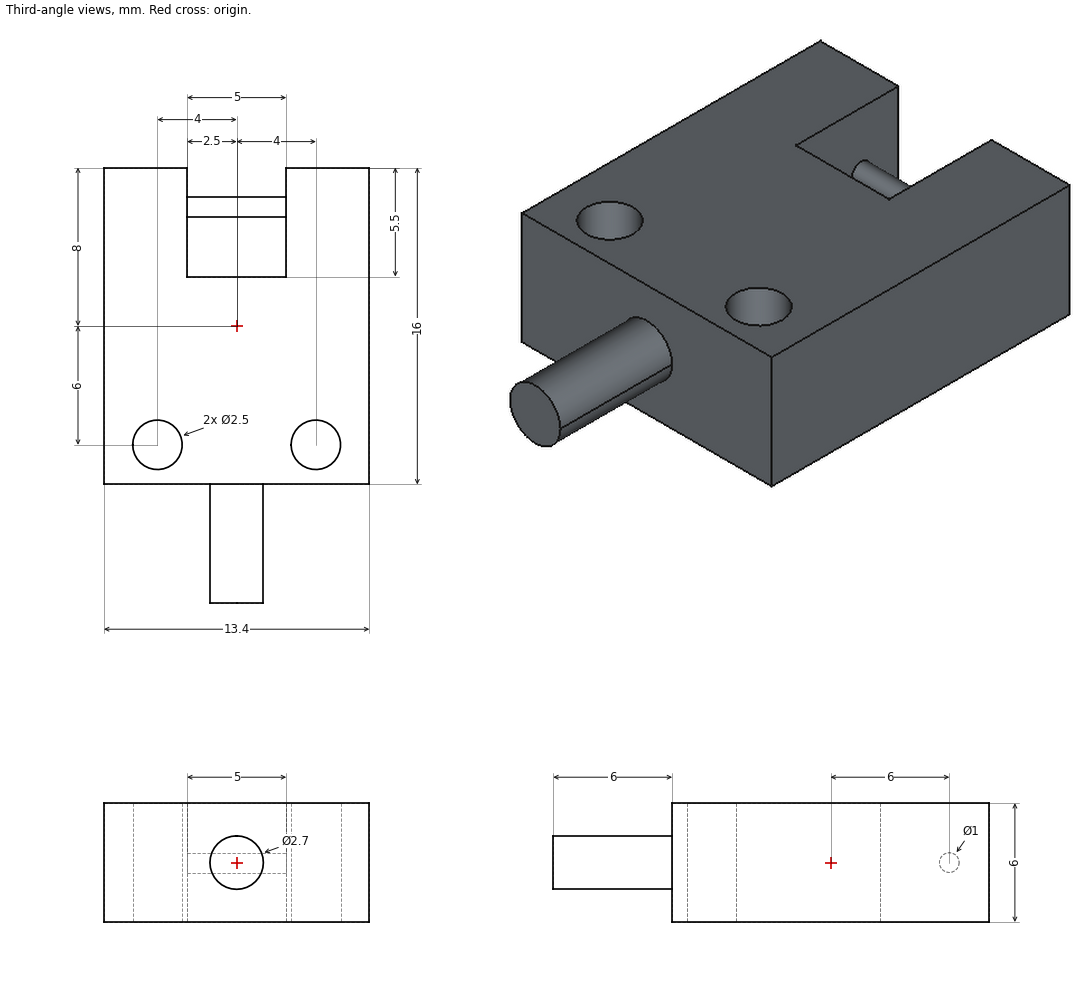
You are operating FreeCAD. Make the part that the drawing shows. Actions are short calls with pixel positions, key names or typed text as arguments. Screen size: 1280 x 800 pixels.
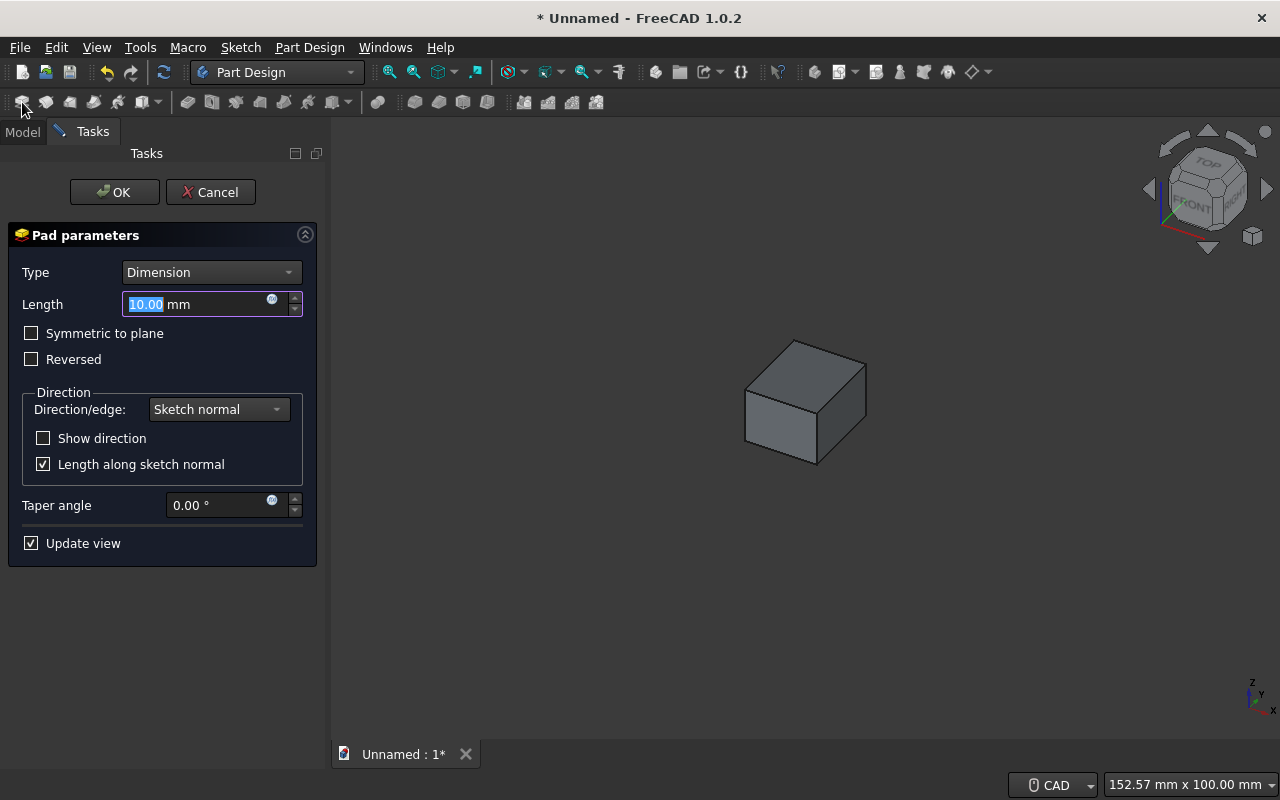
text(6)
key(Tab)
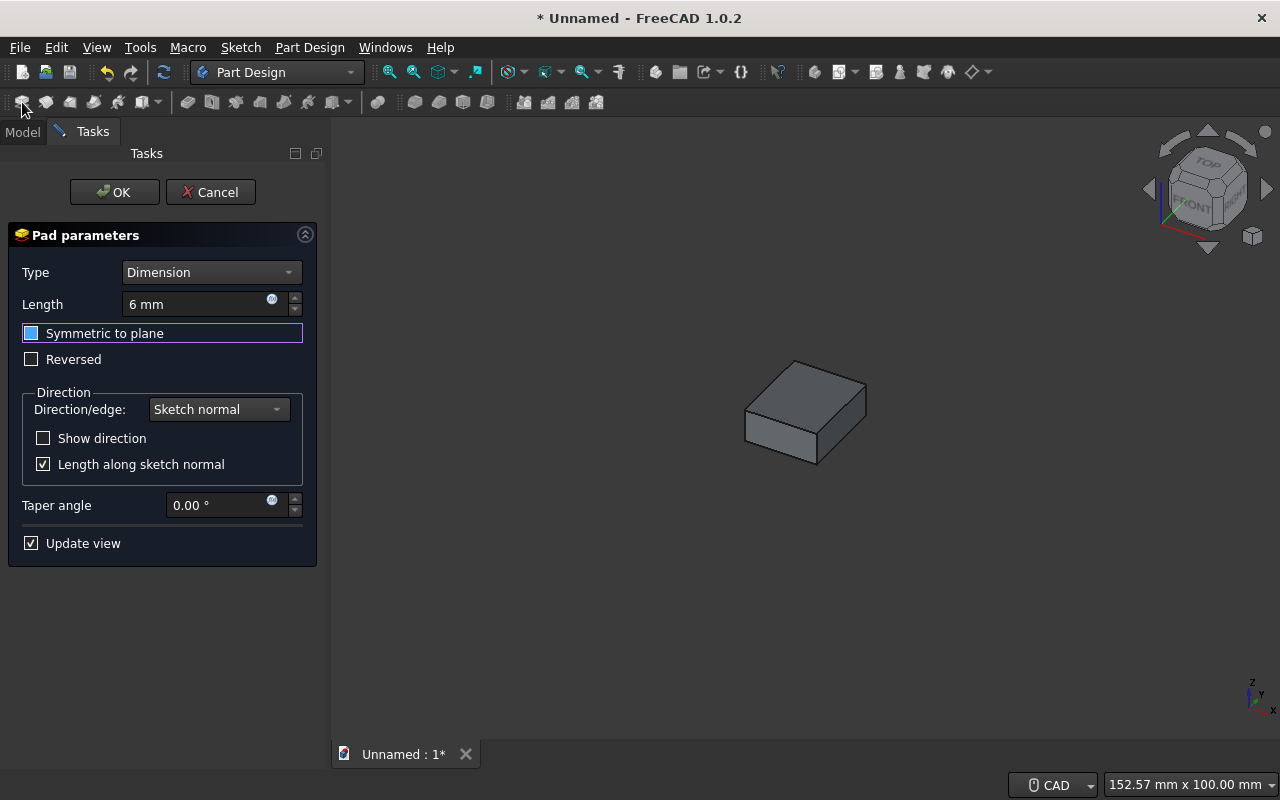
click(30, 333)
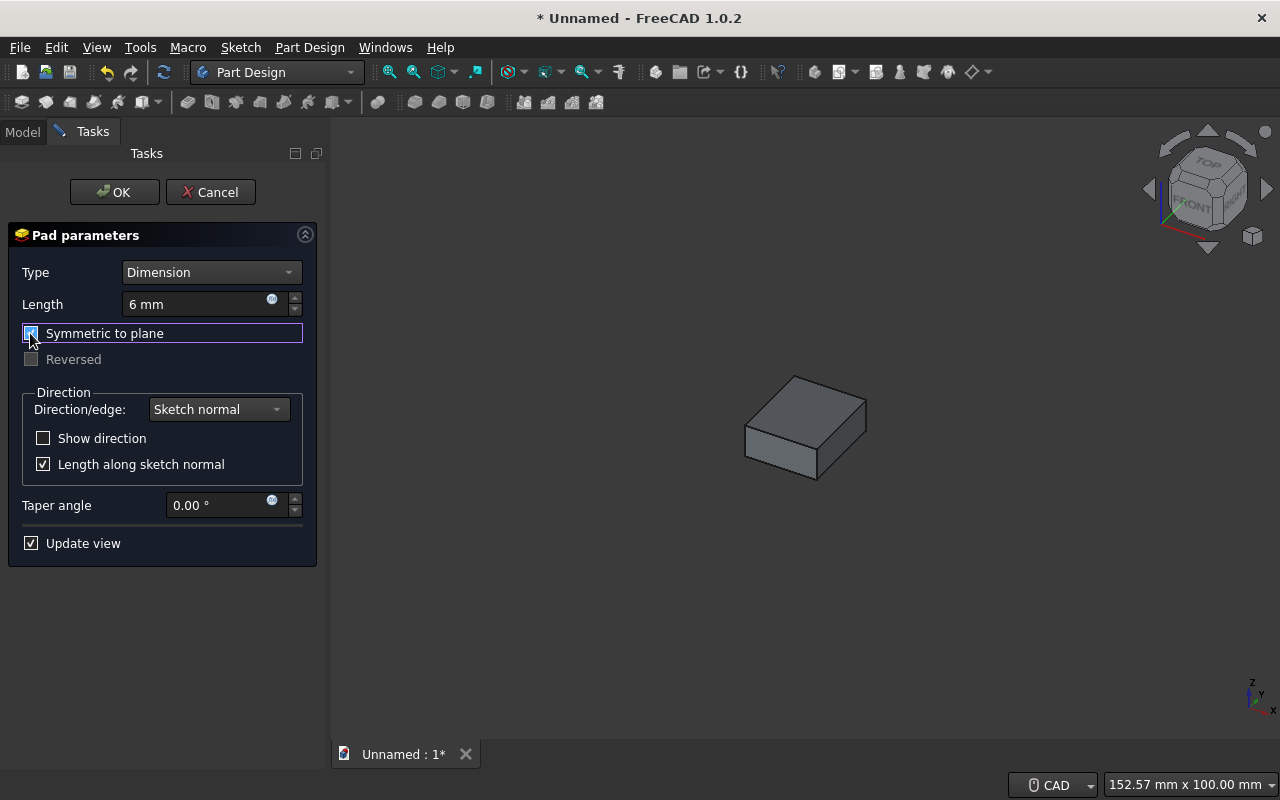
click(115, 192)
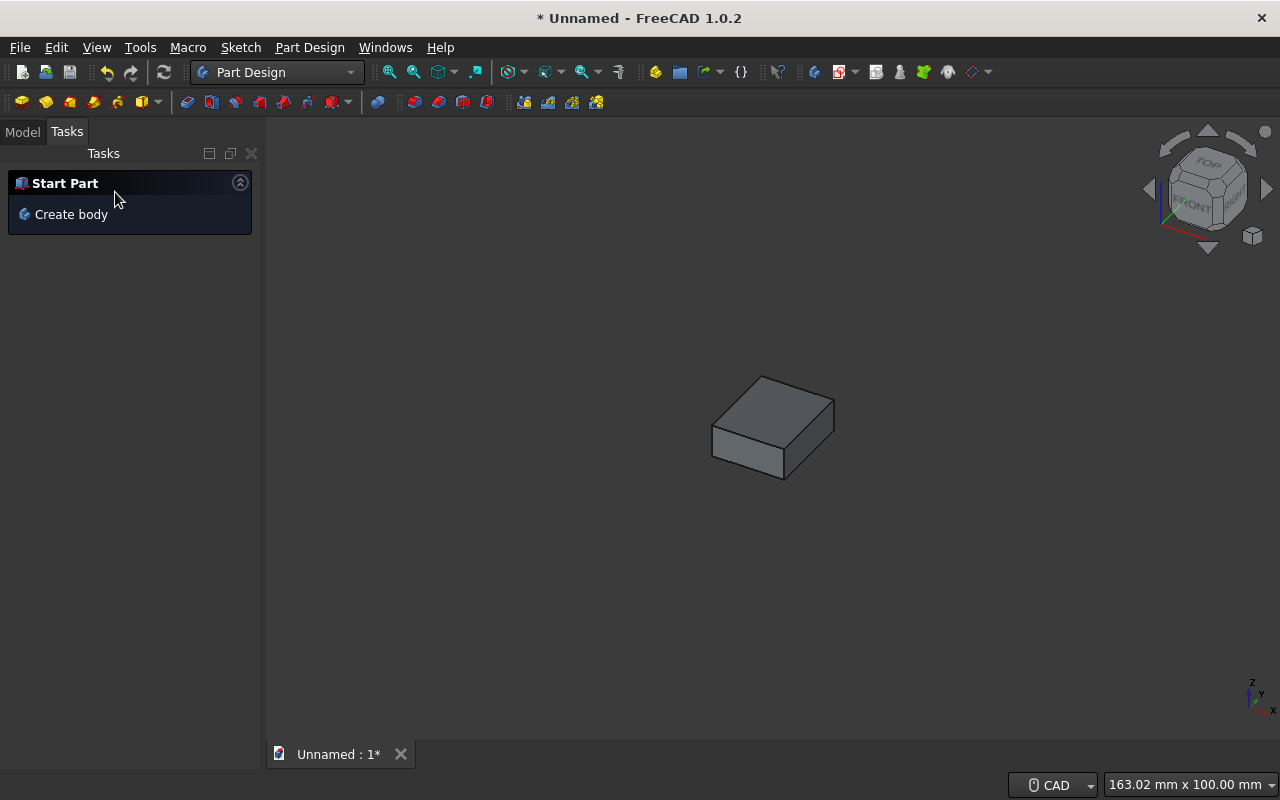
key(v)
key(f)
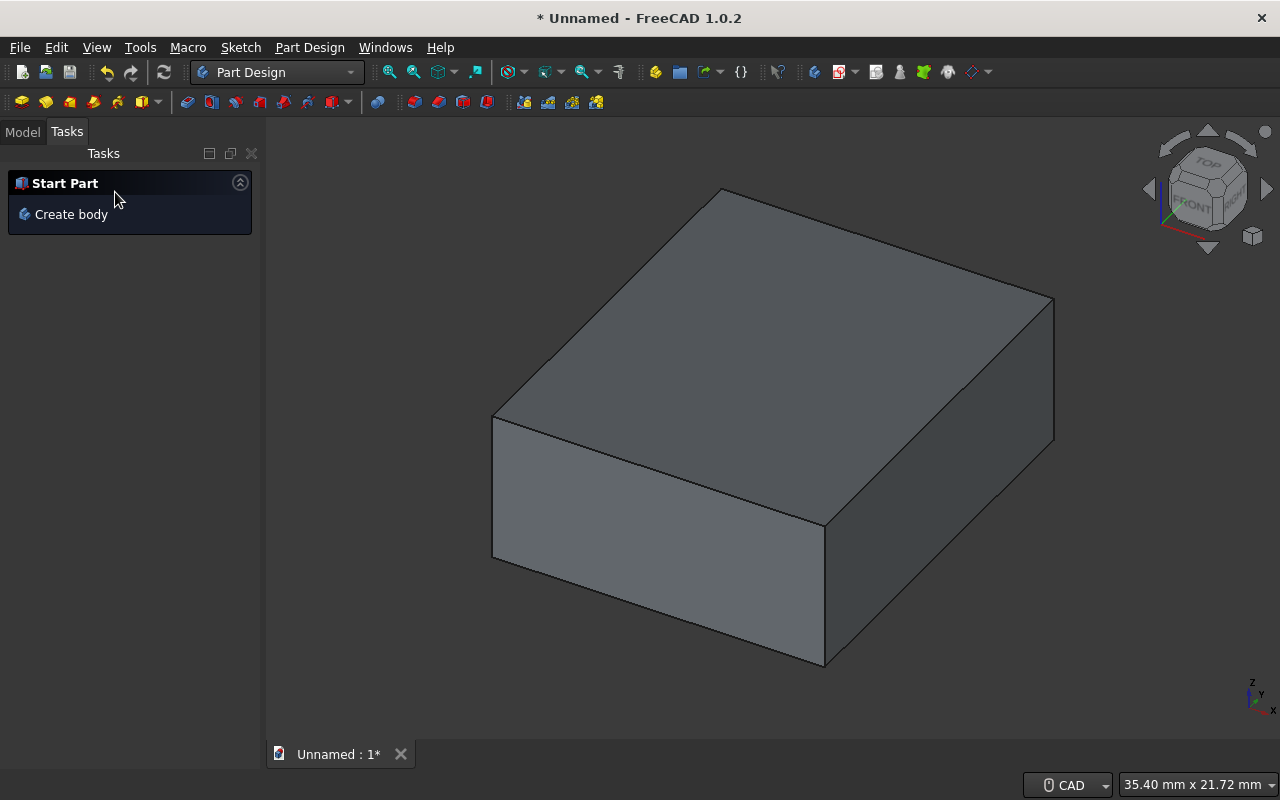
click(773, 357)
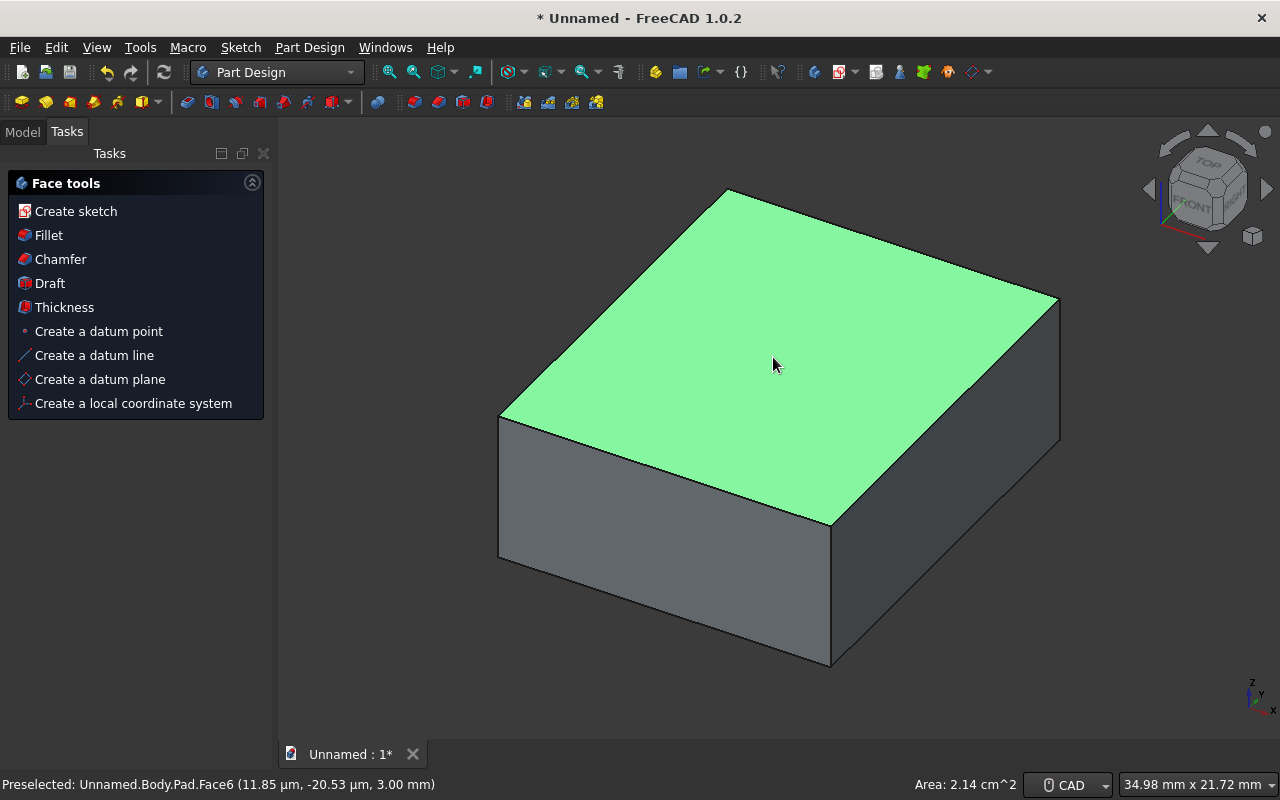
click(840, 72)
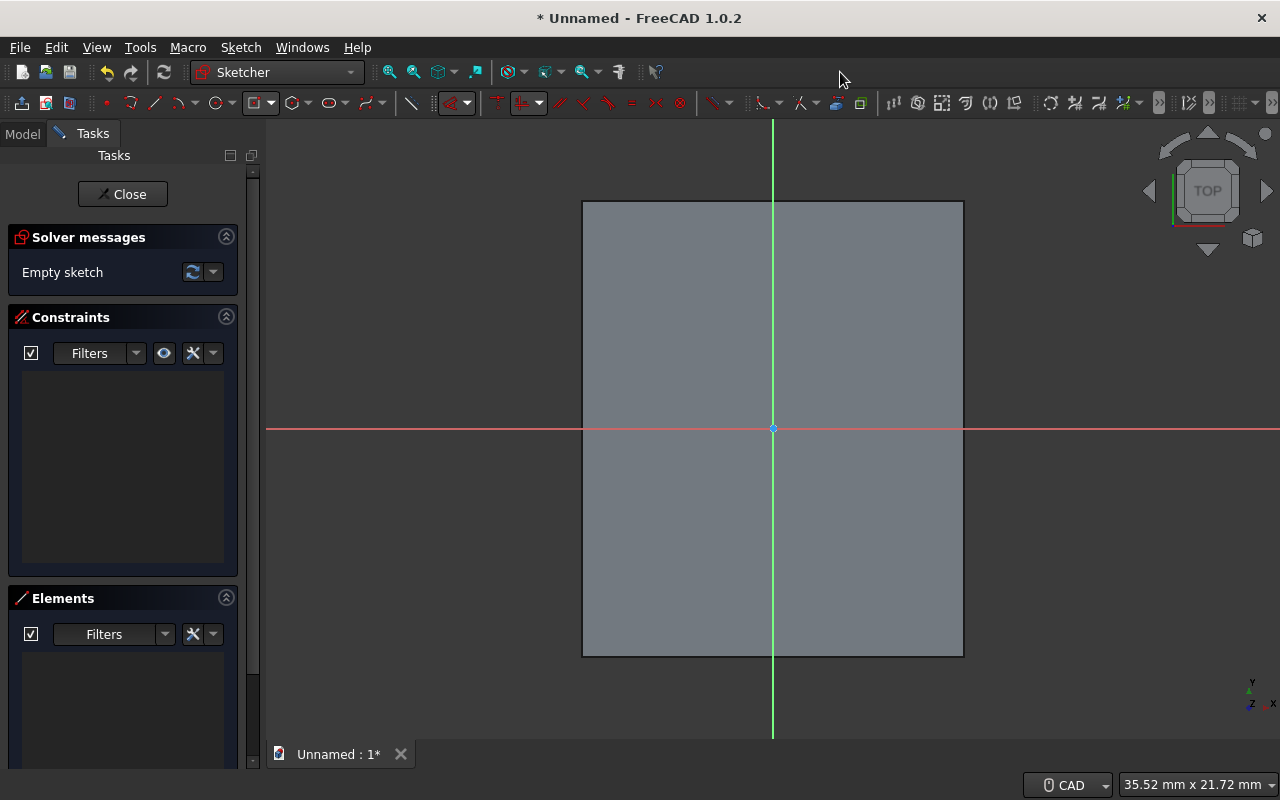
scroll(856, 176, up, 3)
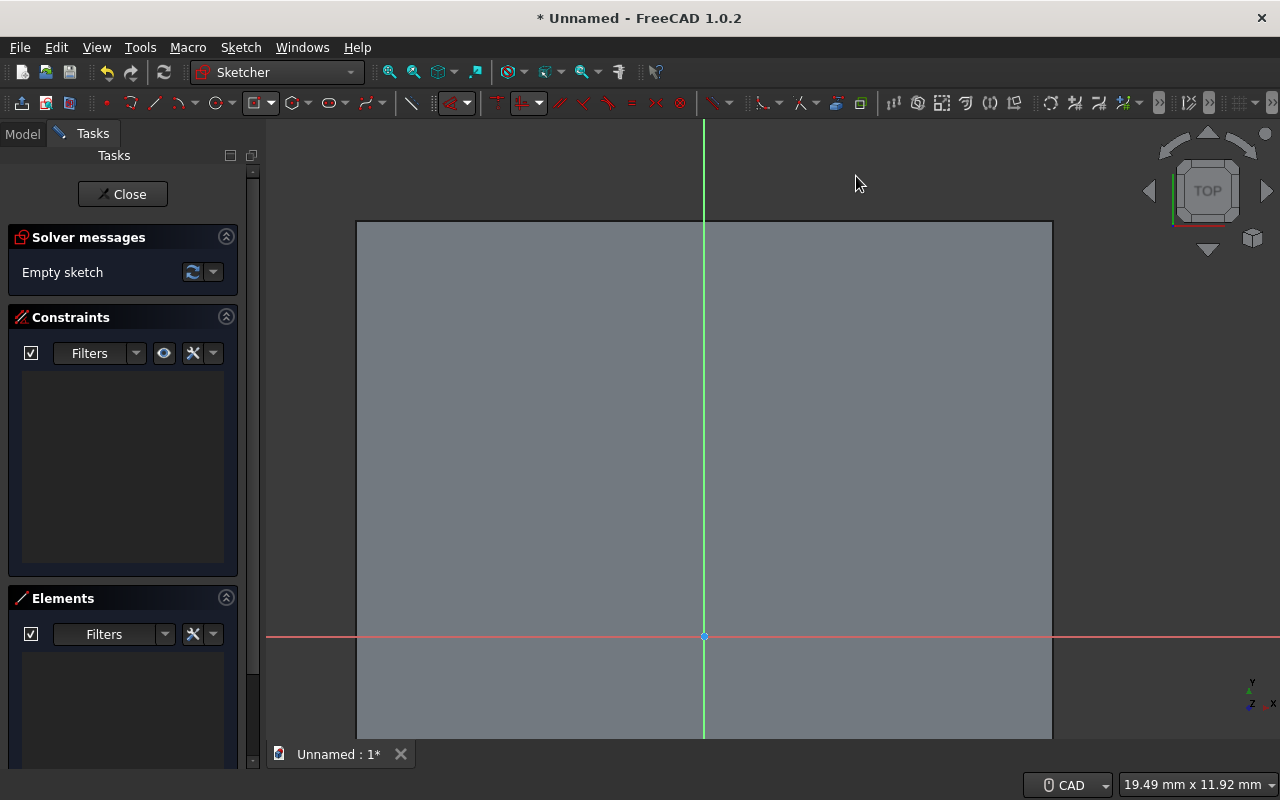
key(g)
key(r)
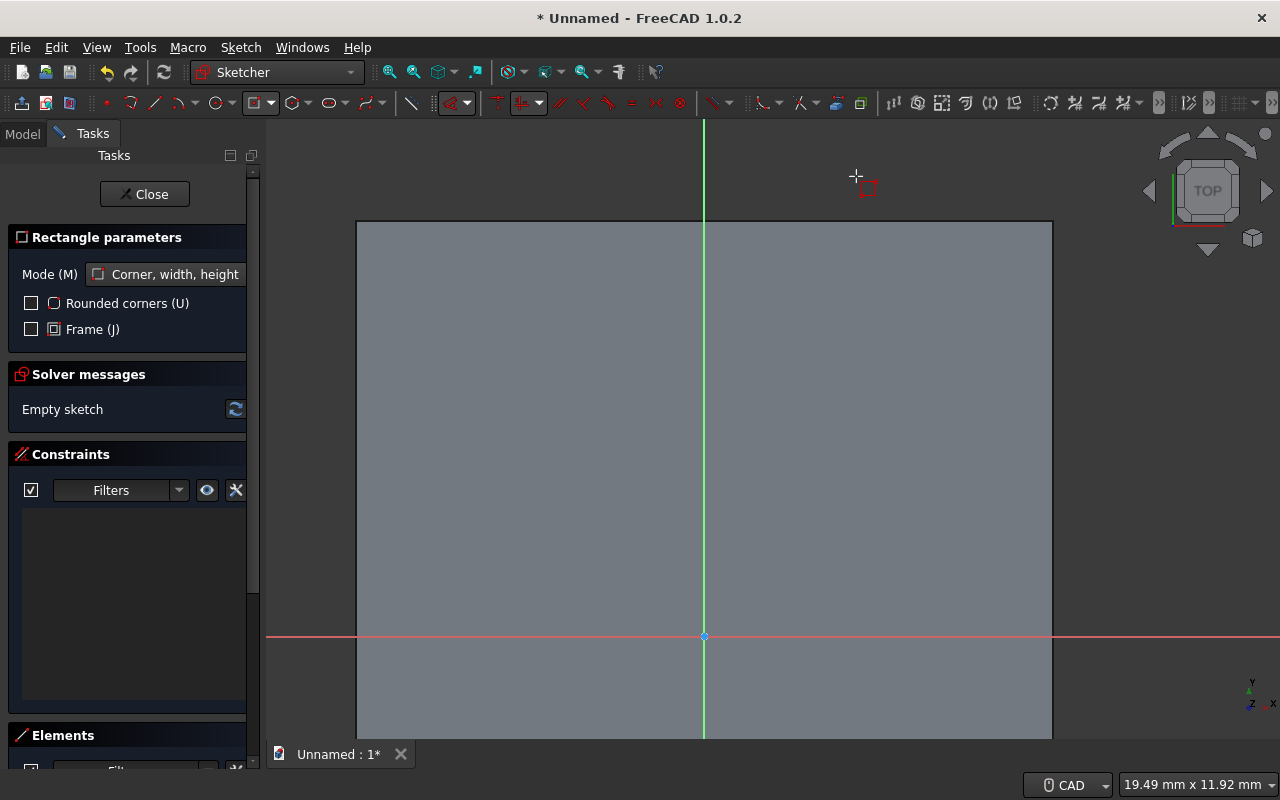
click(574, 221)
move(834, 507)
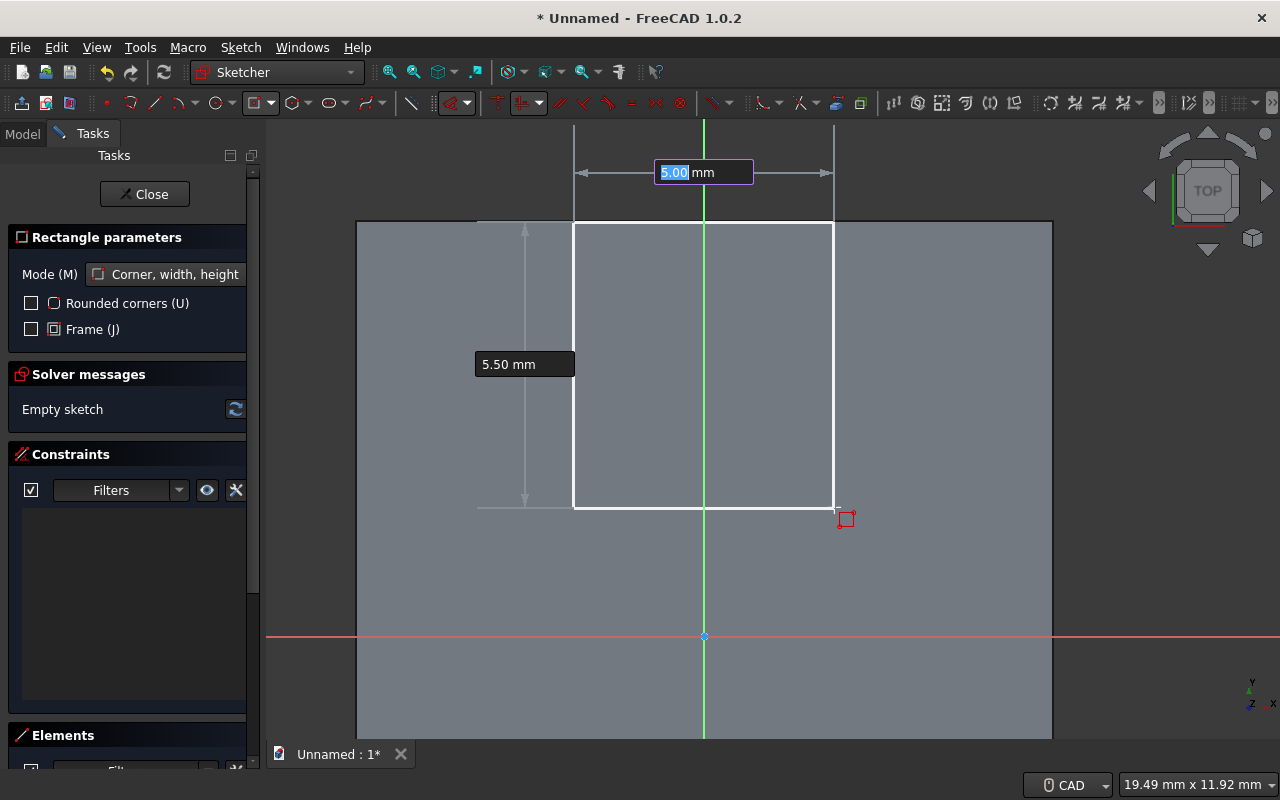
text(5)
key(Tab)
text(5.5)
key(Return)
key(Escape)